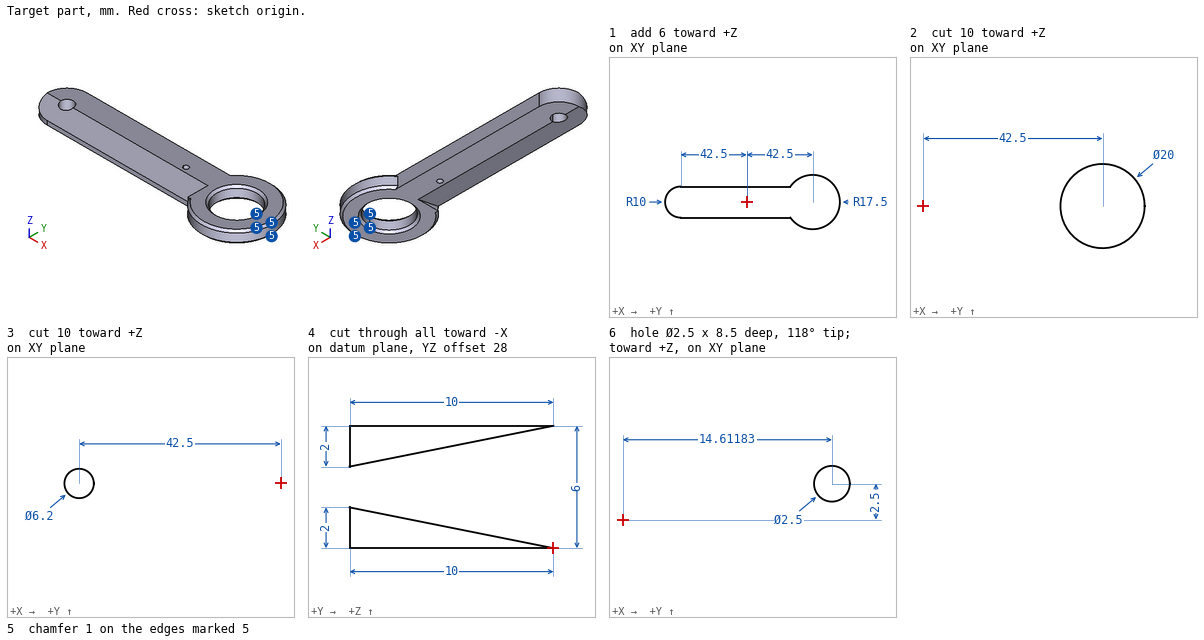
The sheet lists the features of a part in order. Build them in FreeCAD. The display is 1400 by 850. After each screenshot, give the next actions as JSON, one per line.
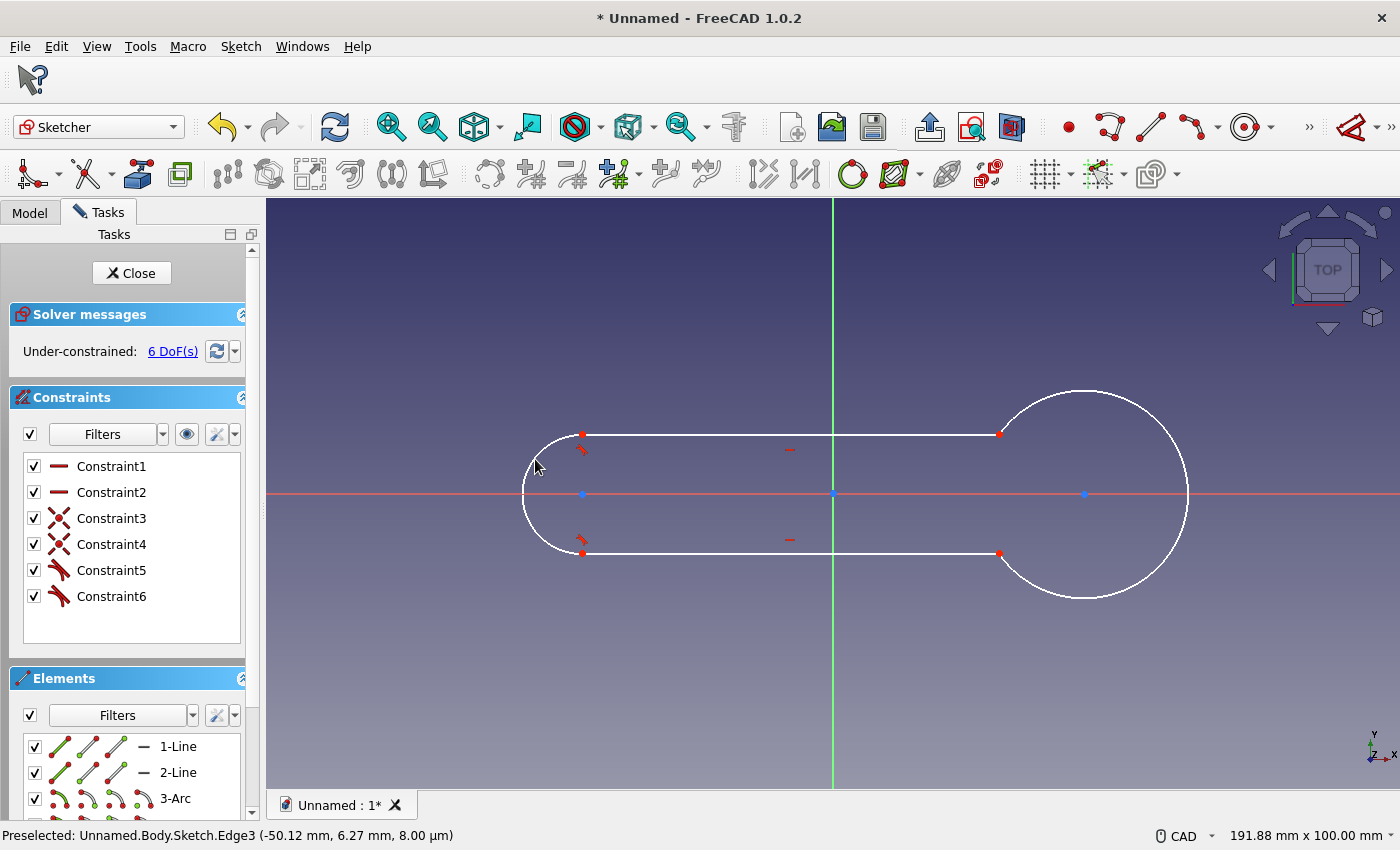
{"action": "left_click", "coordinate": [582, 494]}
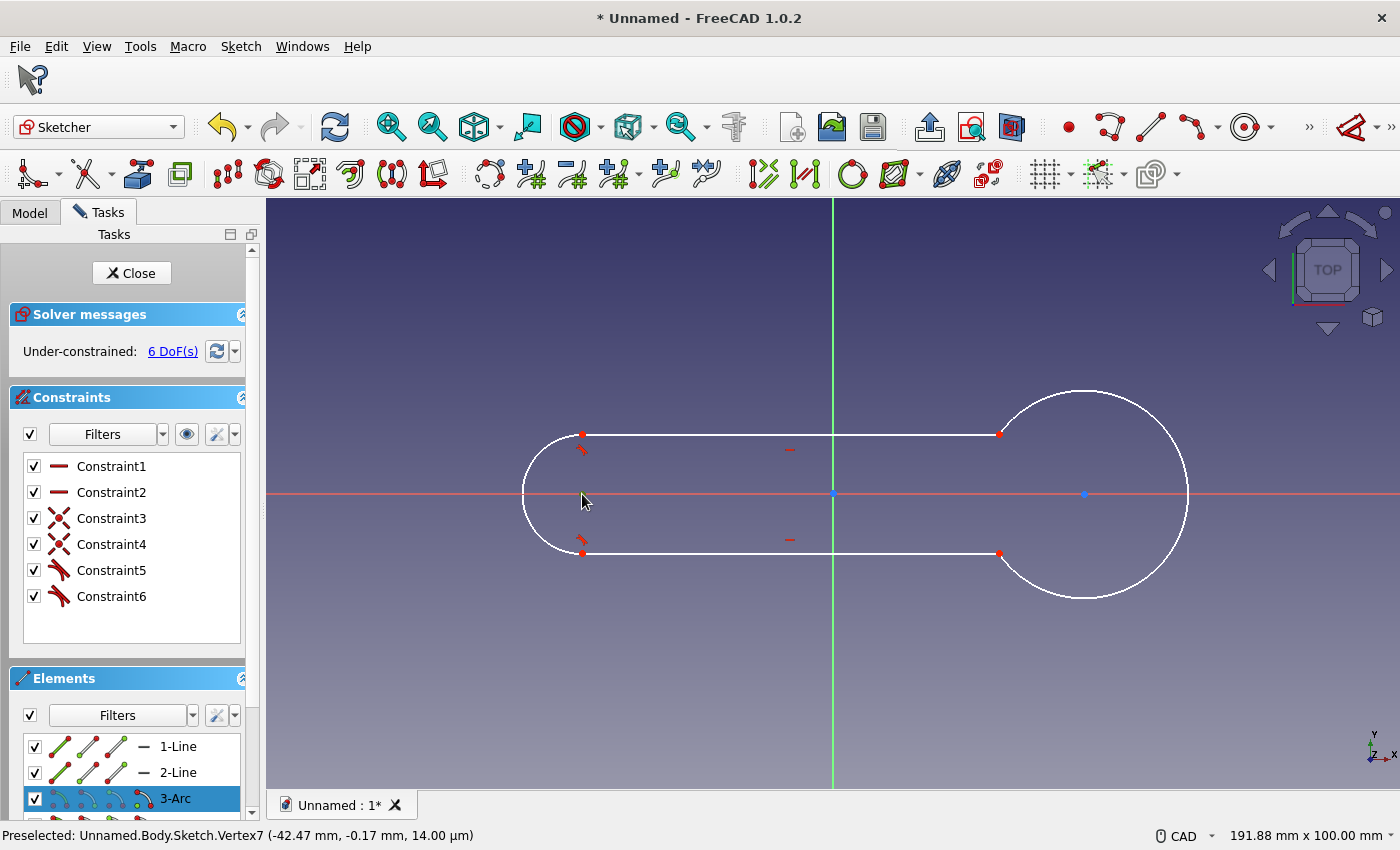
{"action": "left_click", "coordinate": [361, 494]}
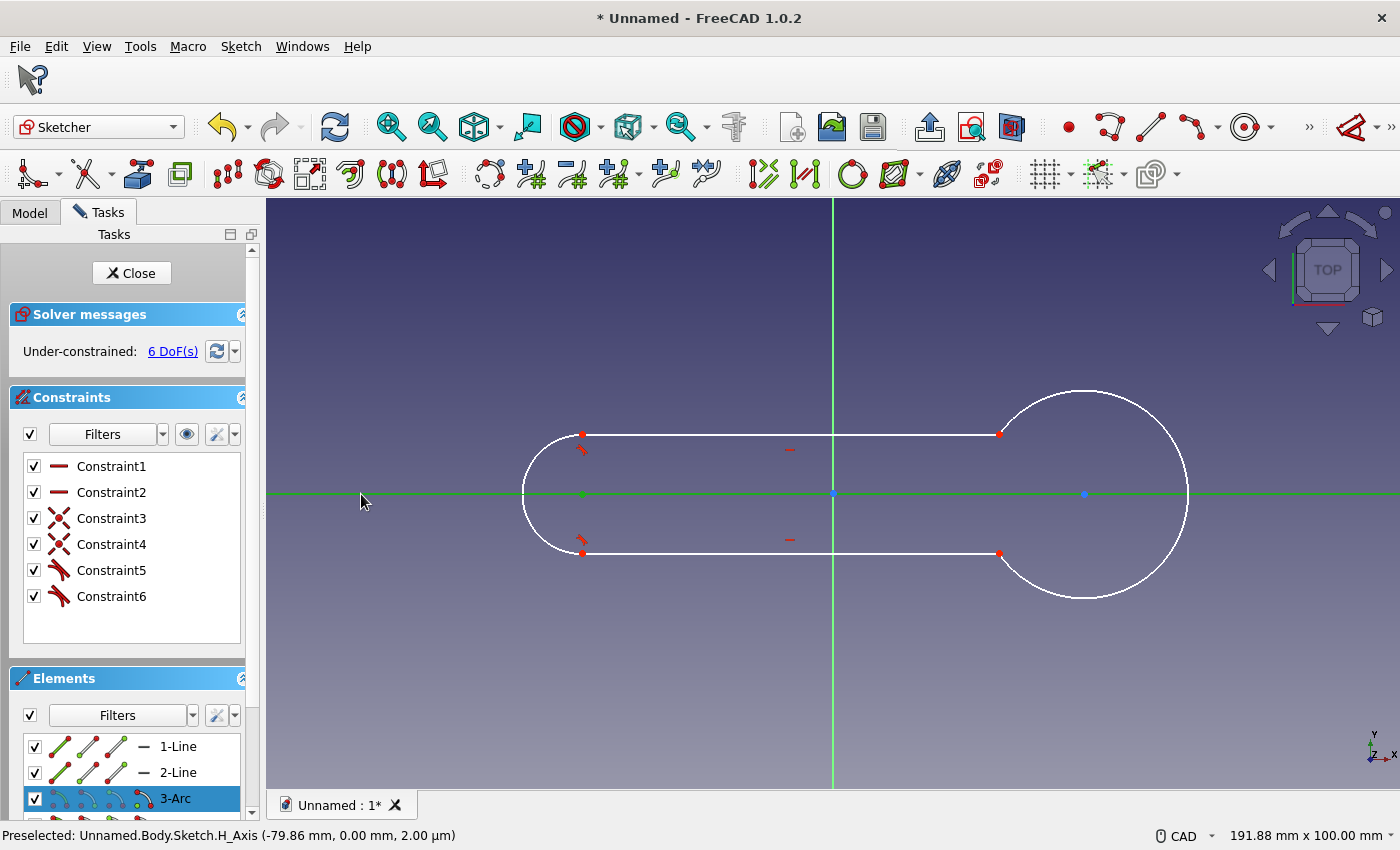
{"action": "key", "text": "c"}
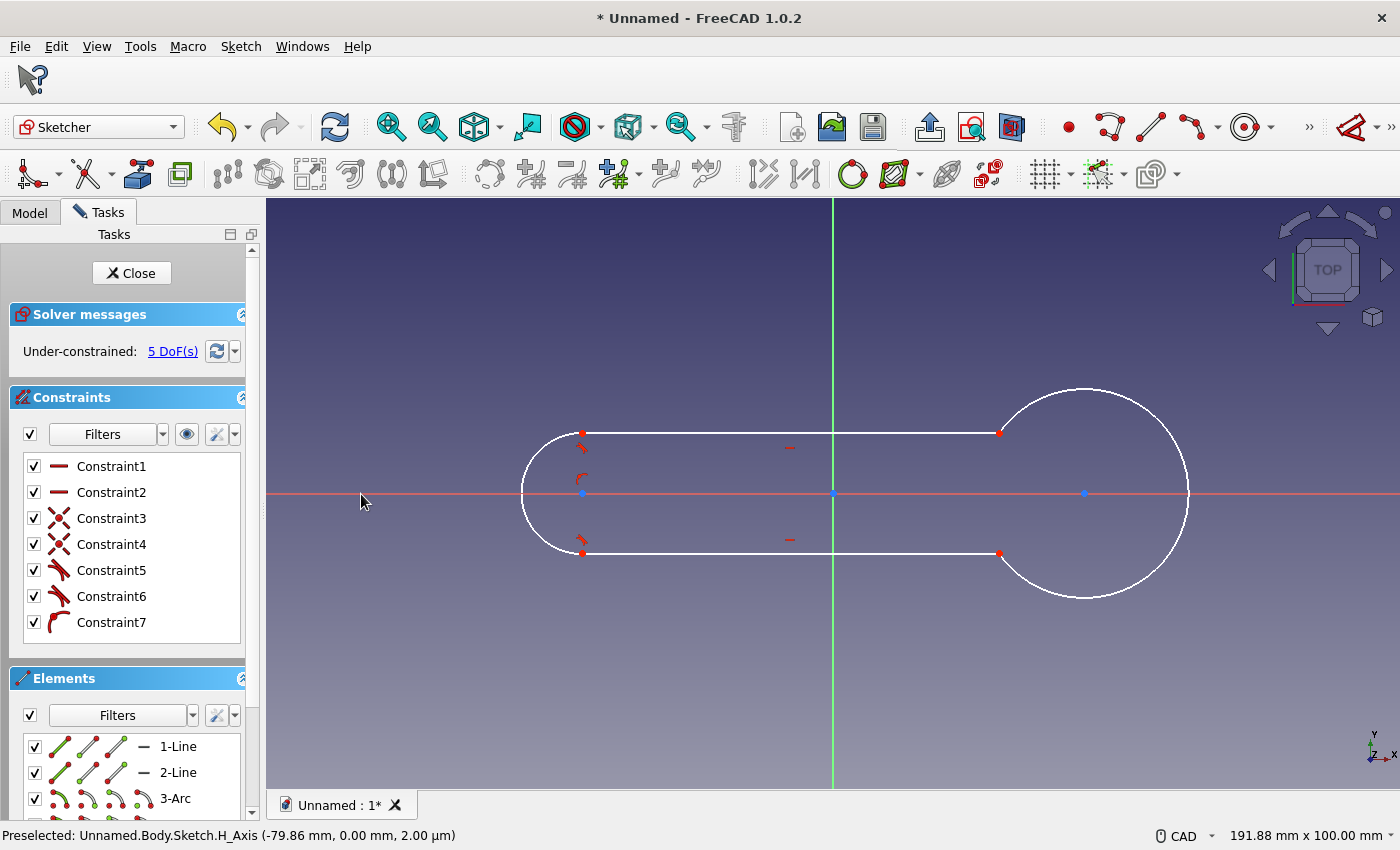
{"action": "left_click", "coordinate": [1084, 493]}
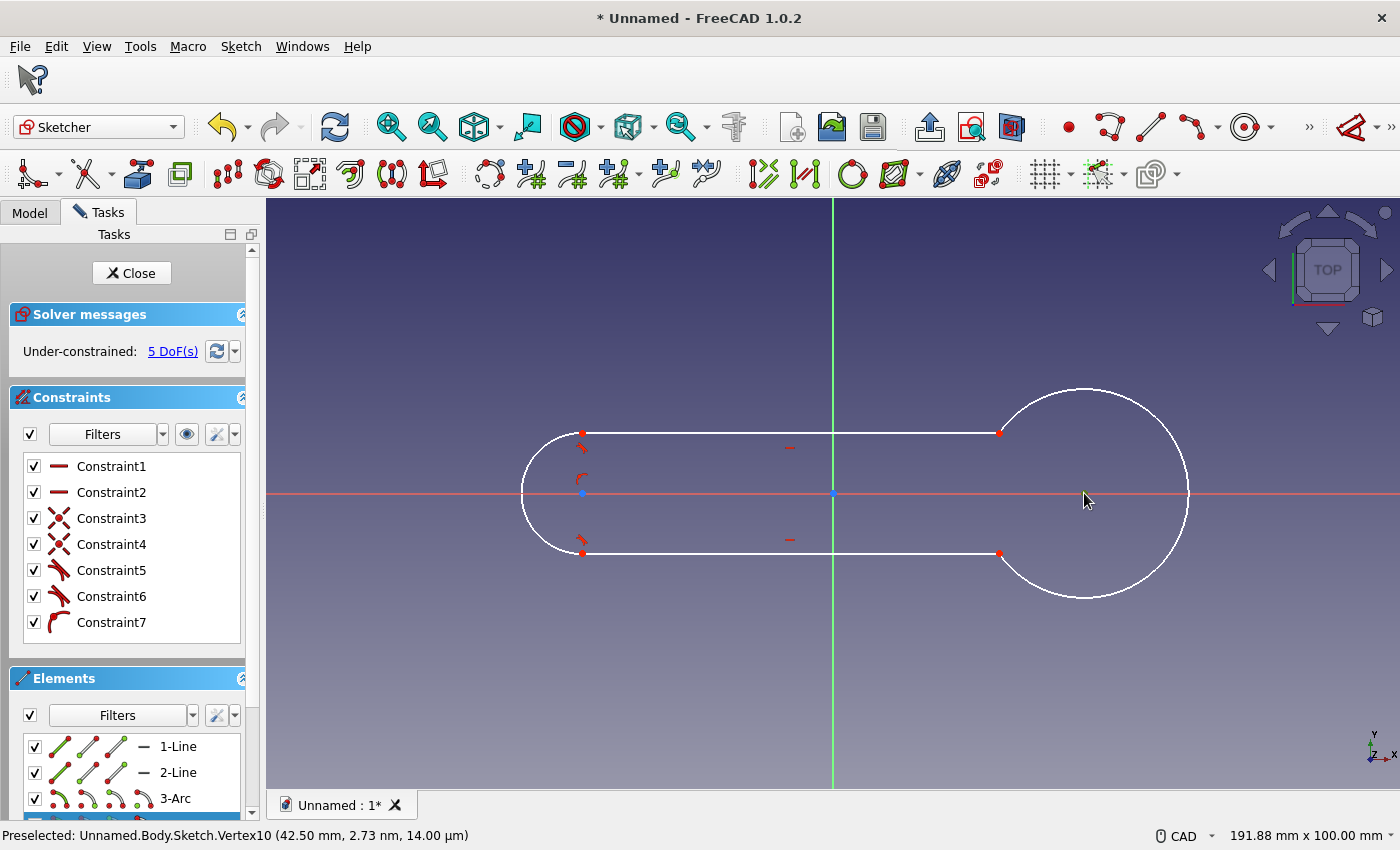
{"action": "left_click", "coordinate": [361, 494]}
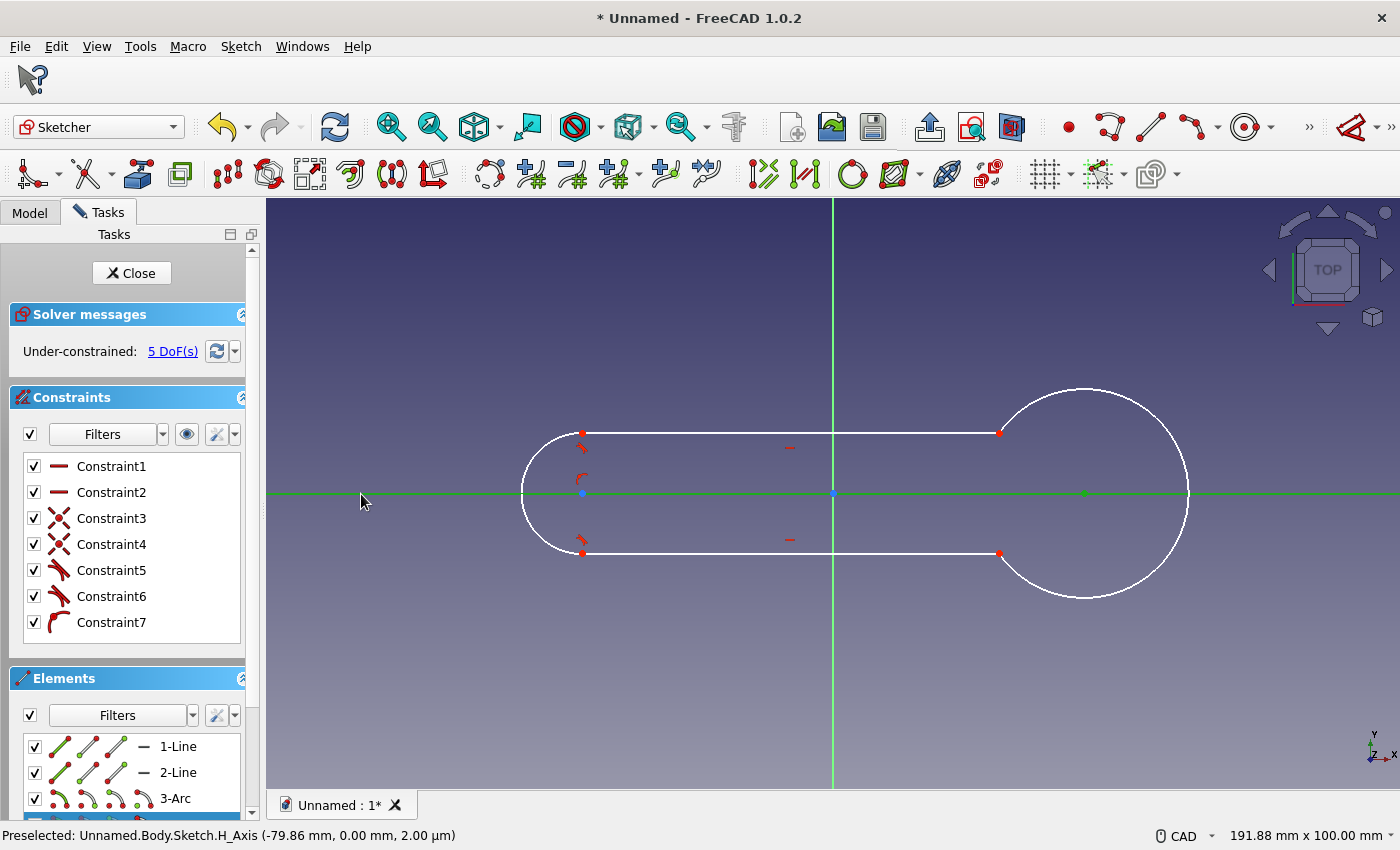
{"action": "key", "text": "c"}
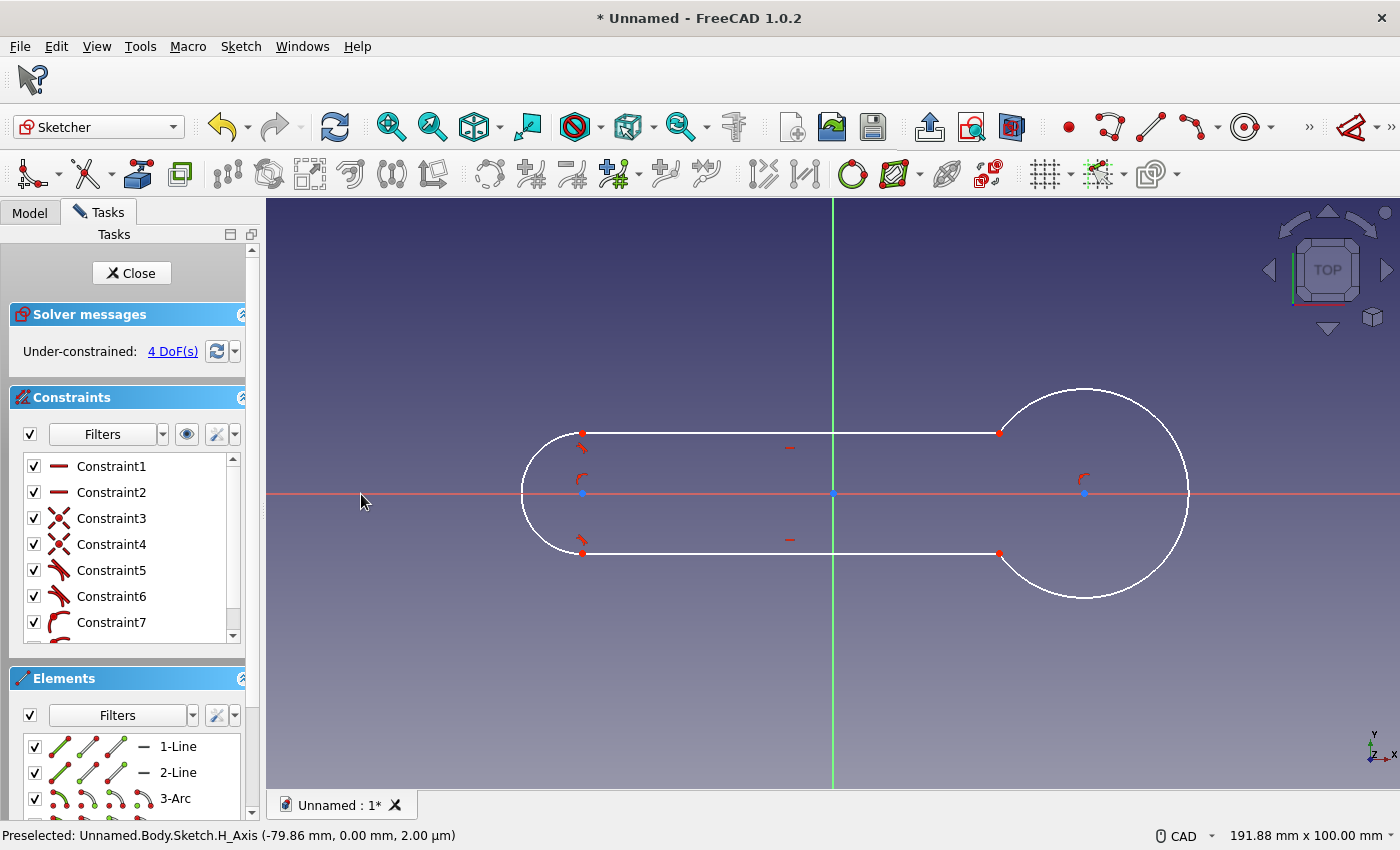
{"action": "key", "text": "d"}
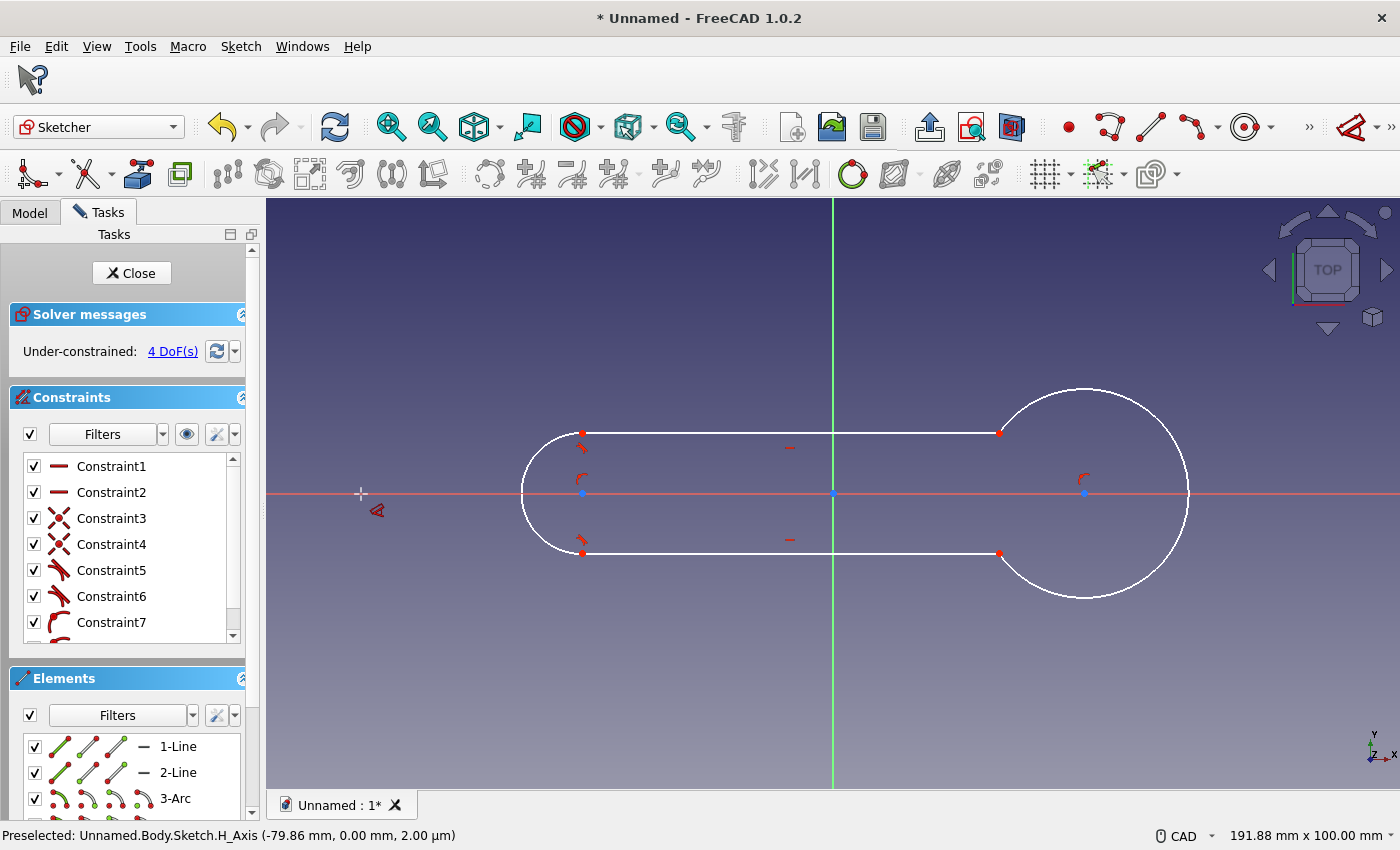
{"action": "left_click", "coordinate": [533, 458]}
{"action": "left_click", "coordinate": [507, 439]}